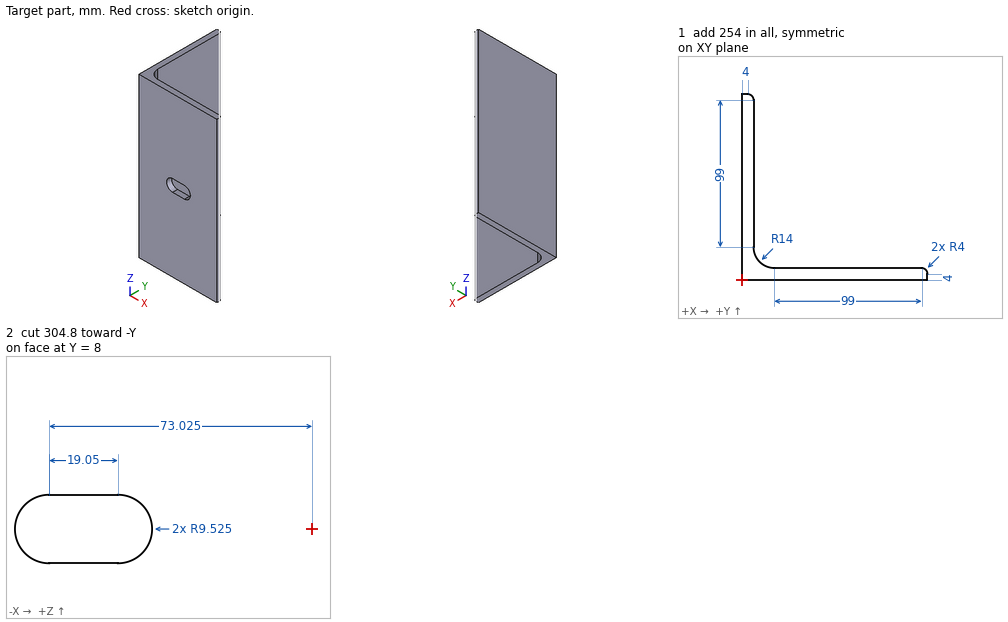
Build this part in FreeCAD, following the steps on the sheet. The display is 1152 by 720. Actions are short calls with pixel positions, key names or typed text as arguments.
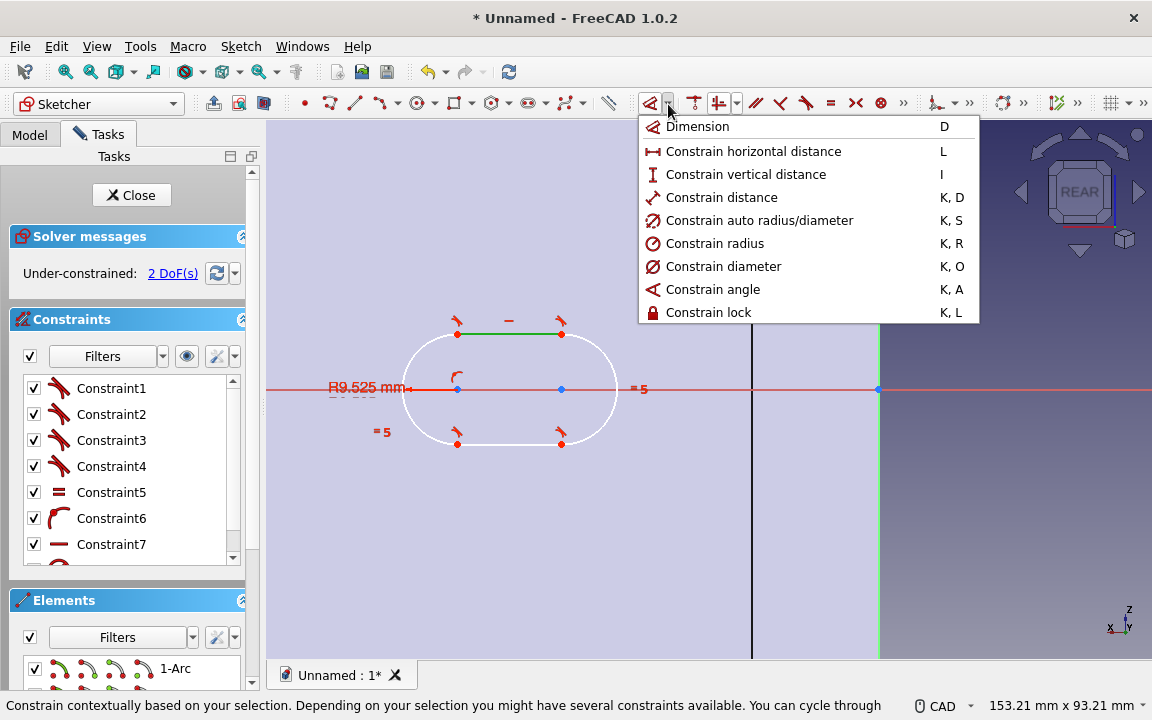
click(809, 152)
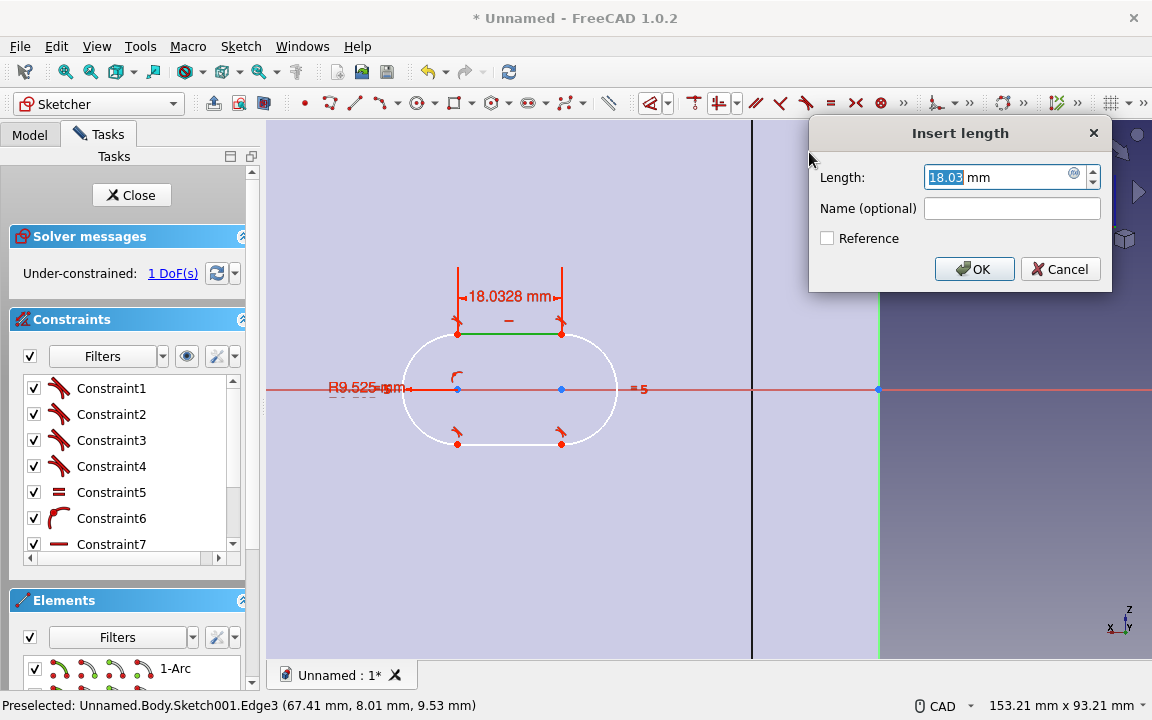
text(19.05)
key(Return)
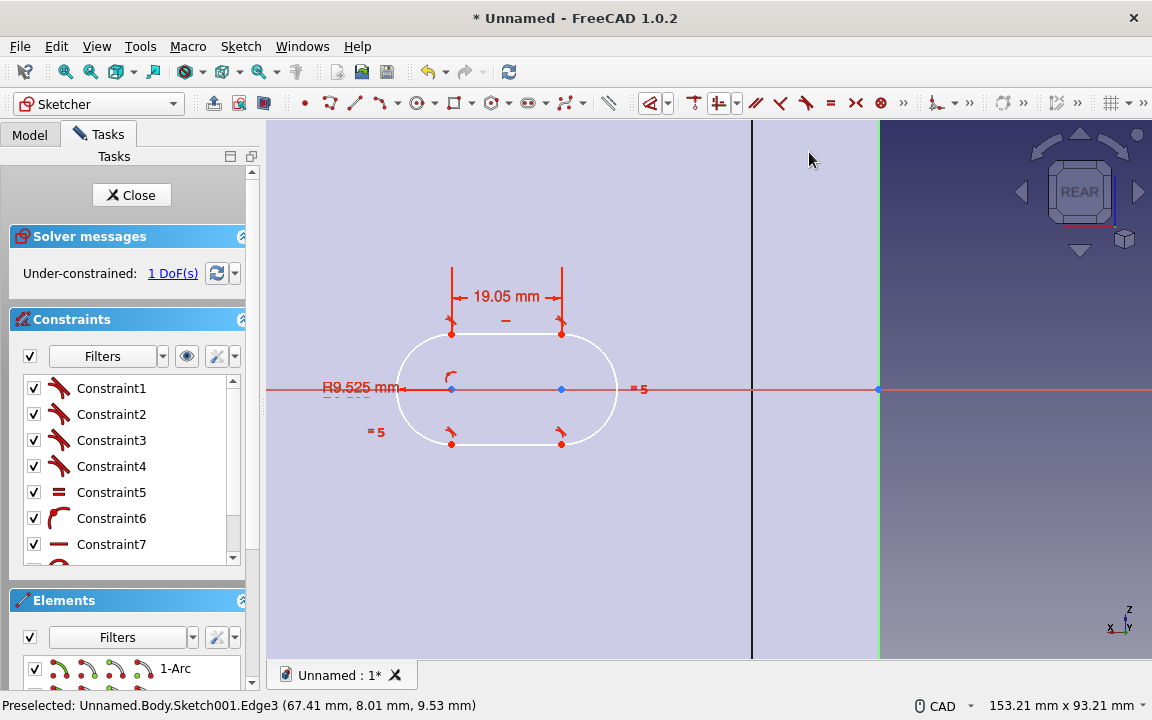
click(452, 334)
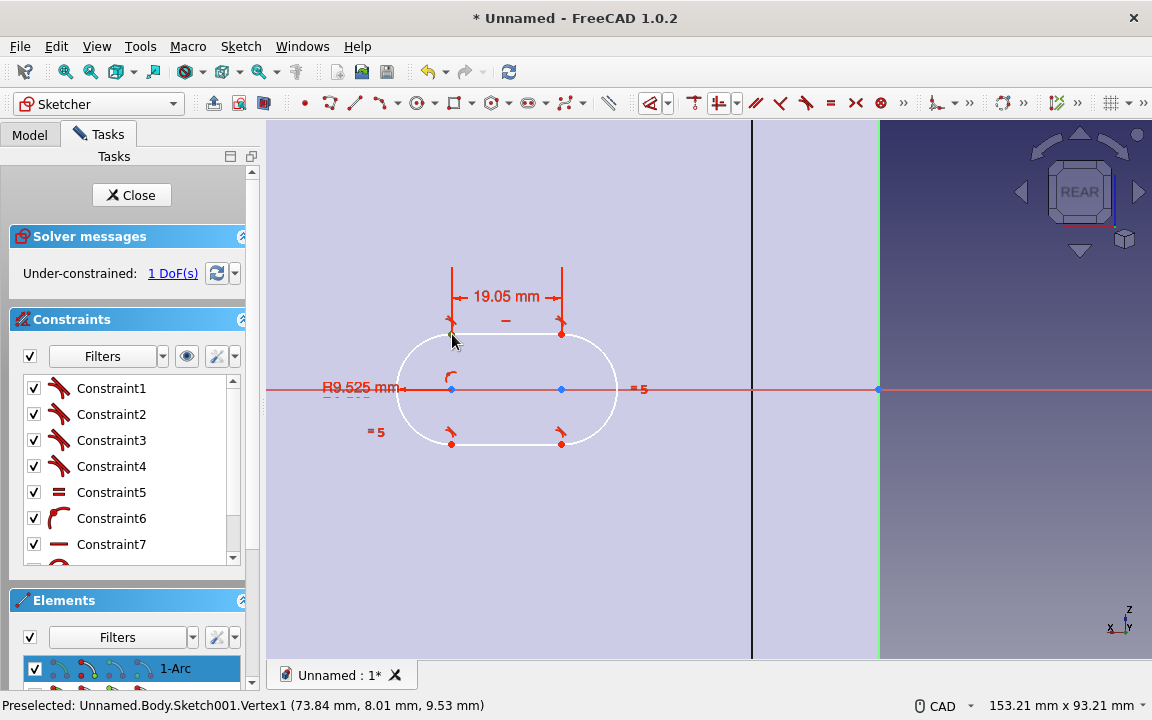
key(l)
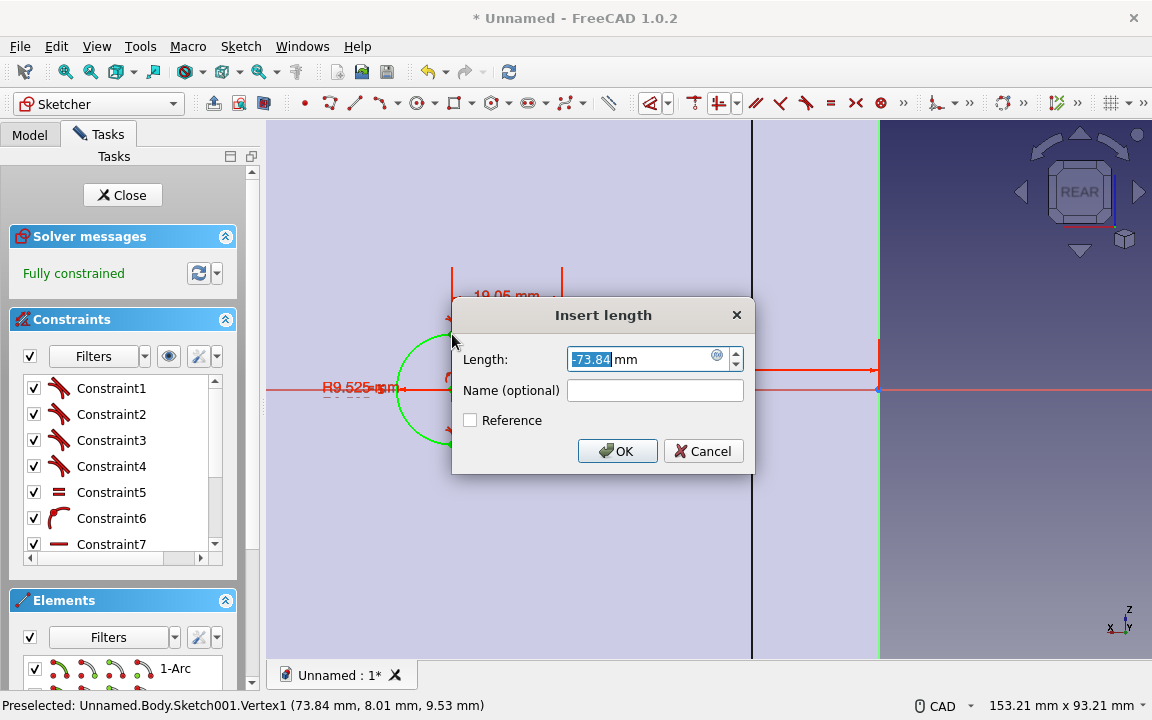
text(-73.025)
key(Return)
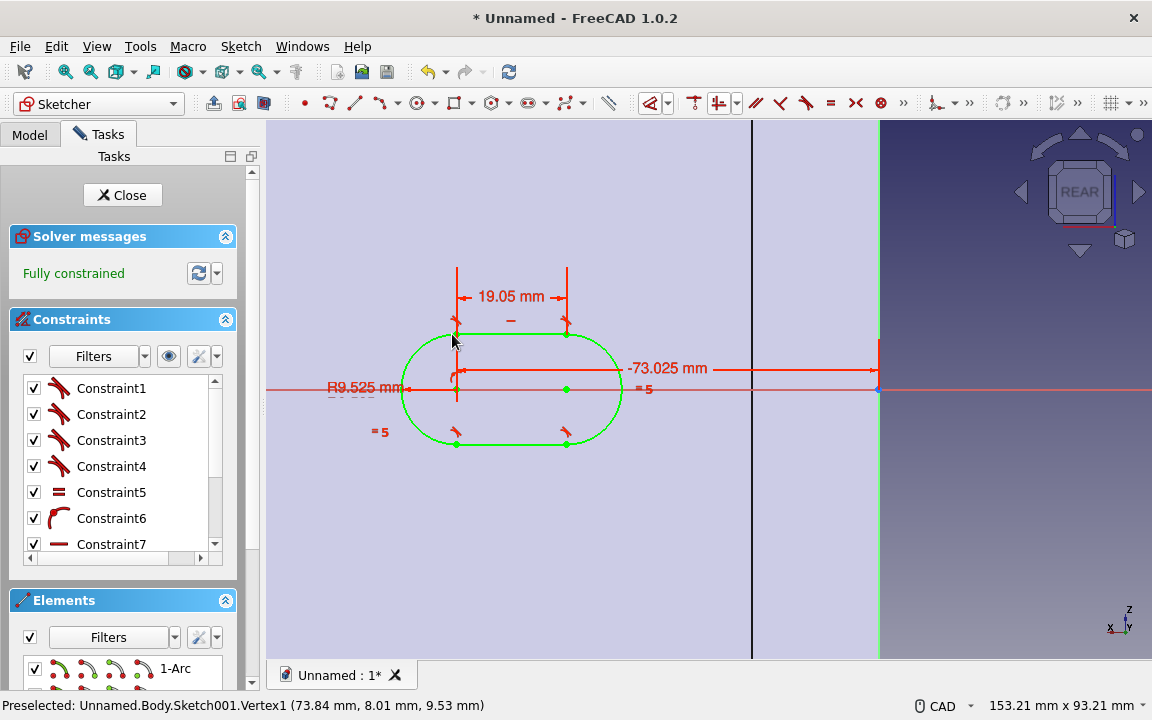
click(123, 195)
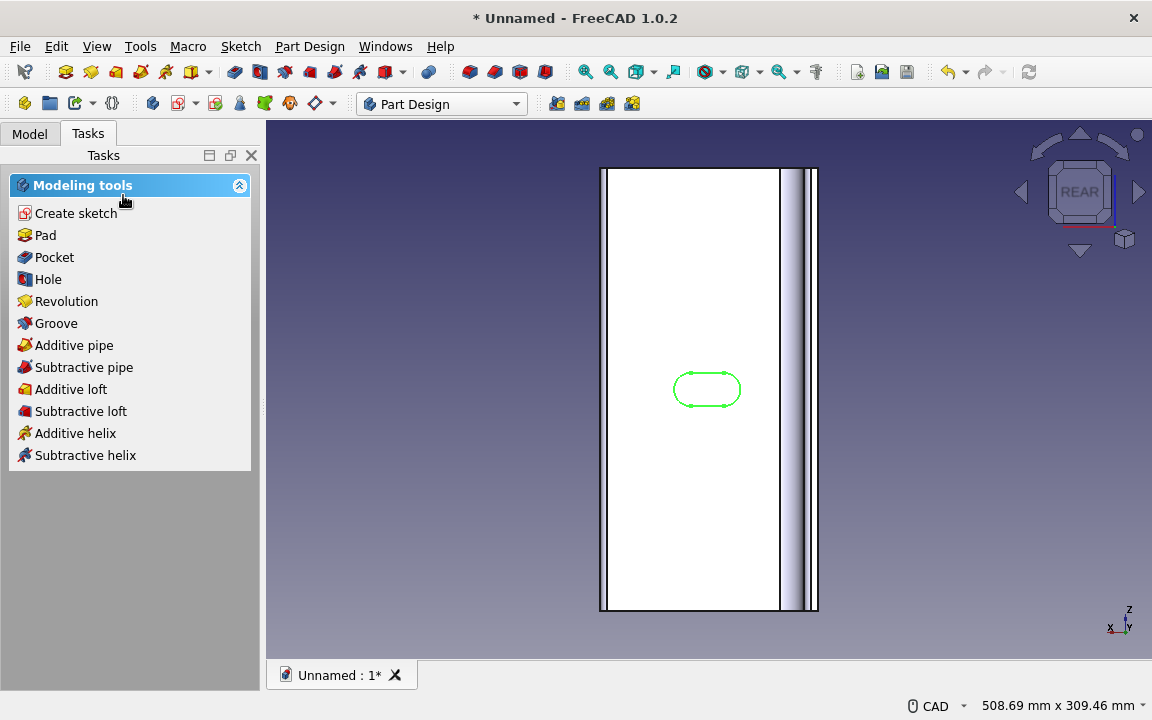
click(235, 72)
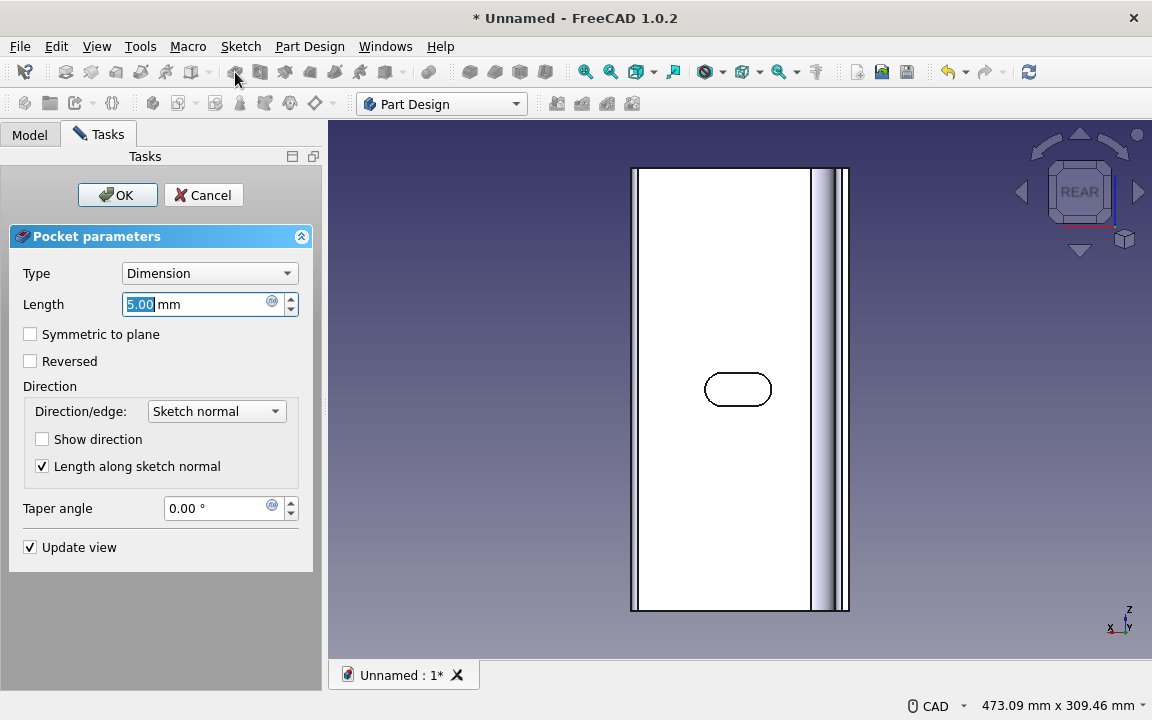
text(304.8)
key(Tab)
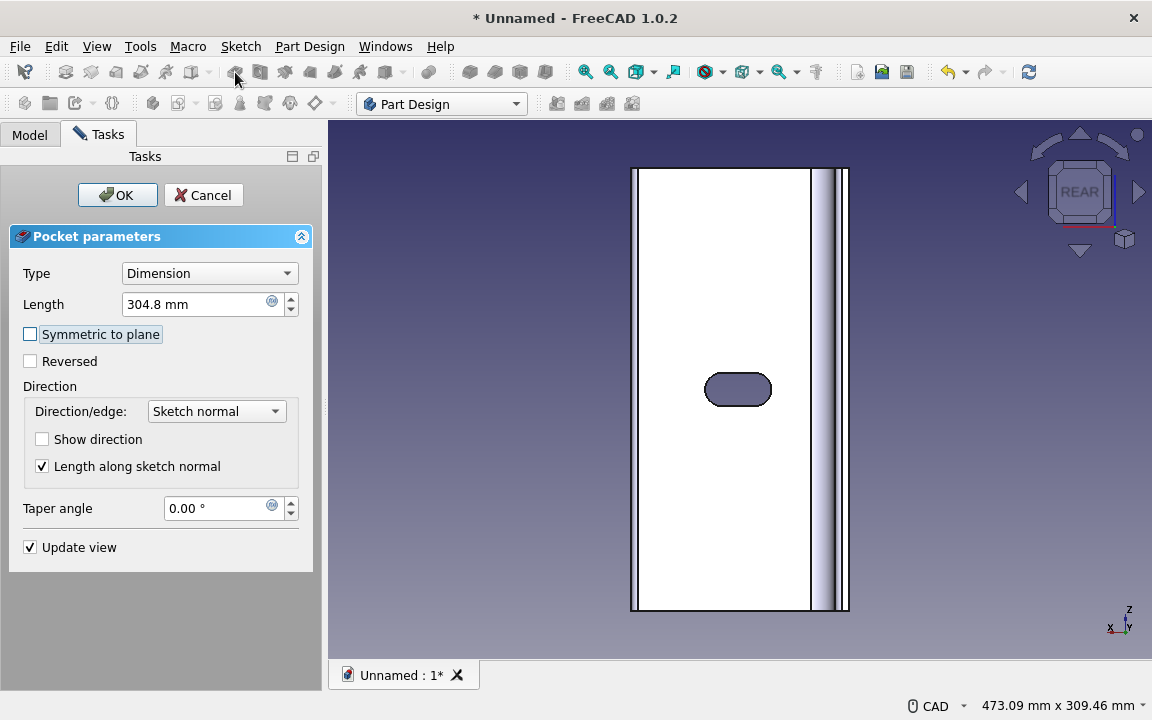
click(118, 195)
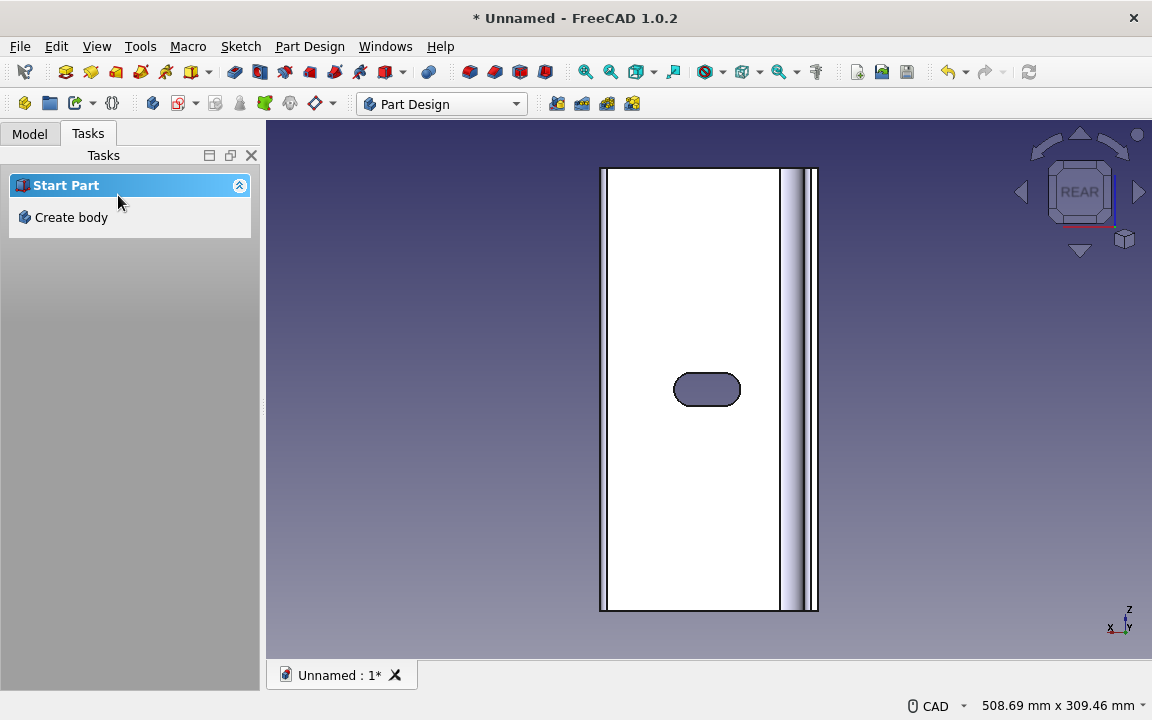
key(0)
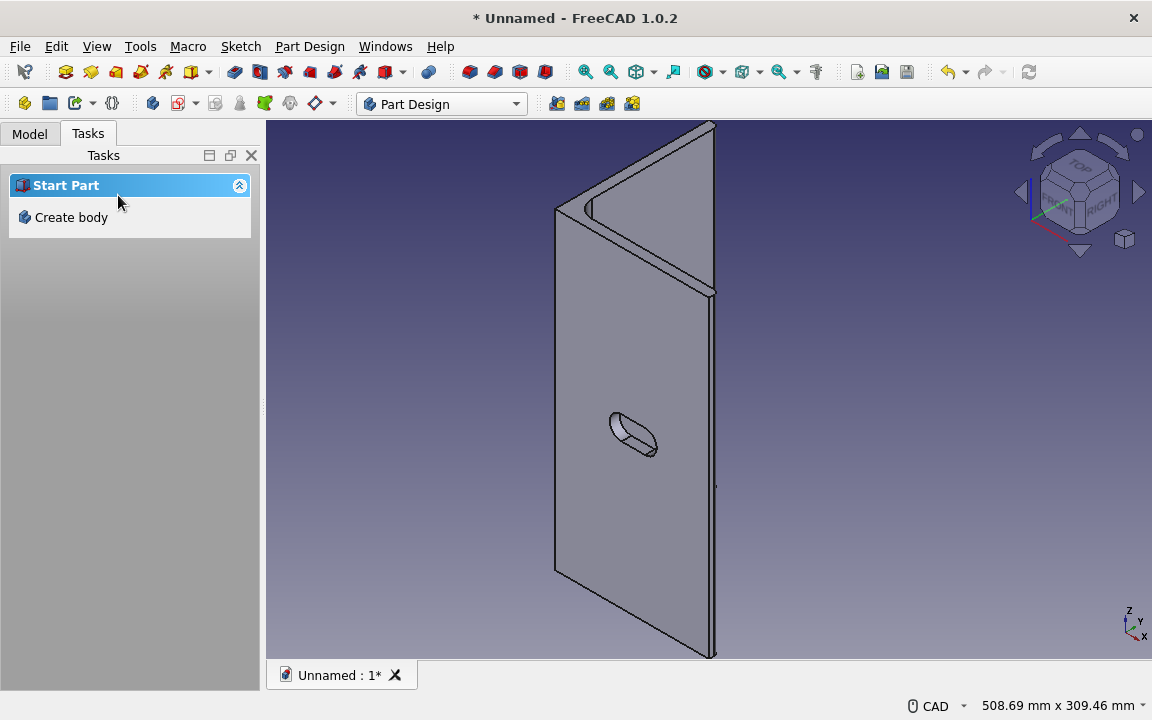
click(586, 72)